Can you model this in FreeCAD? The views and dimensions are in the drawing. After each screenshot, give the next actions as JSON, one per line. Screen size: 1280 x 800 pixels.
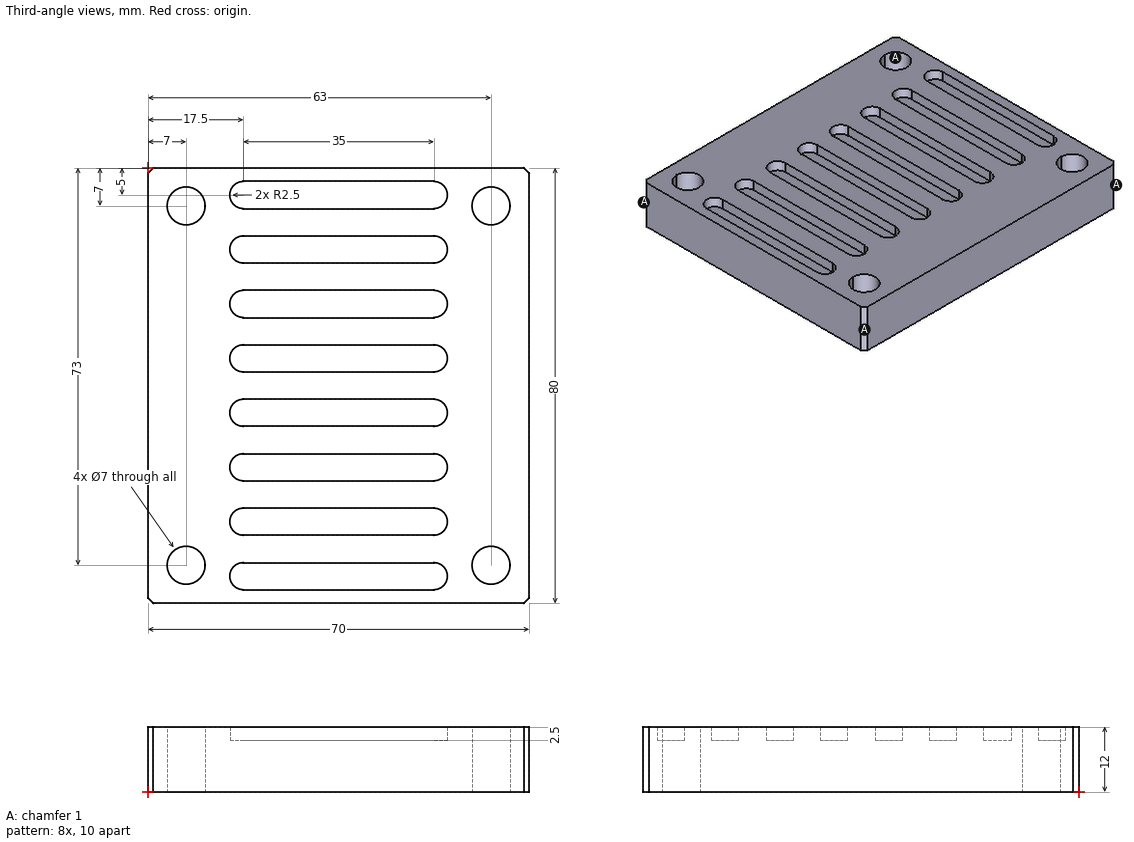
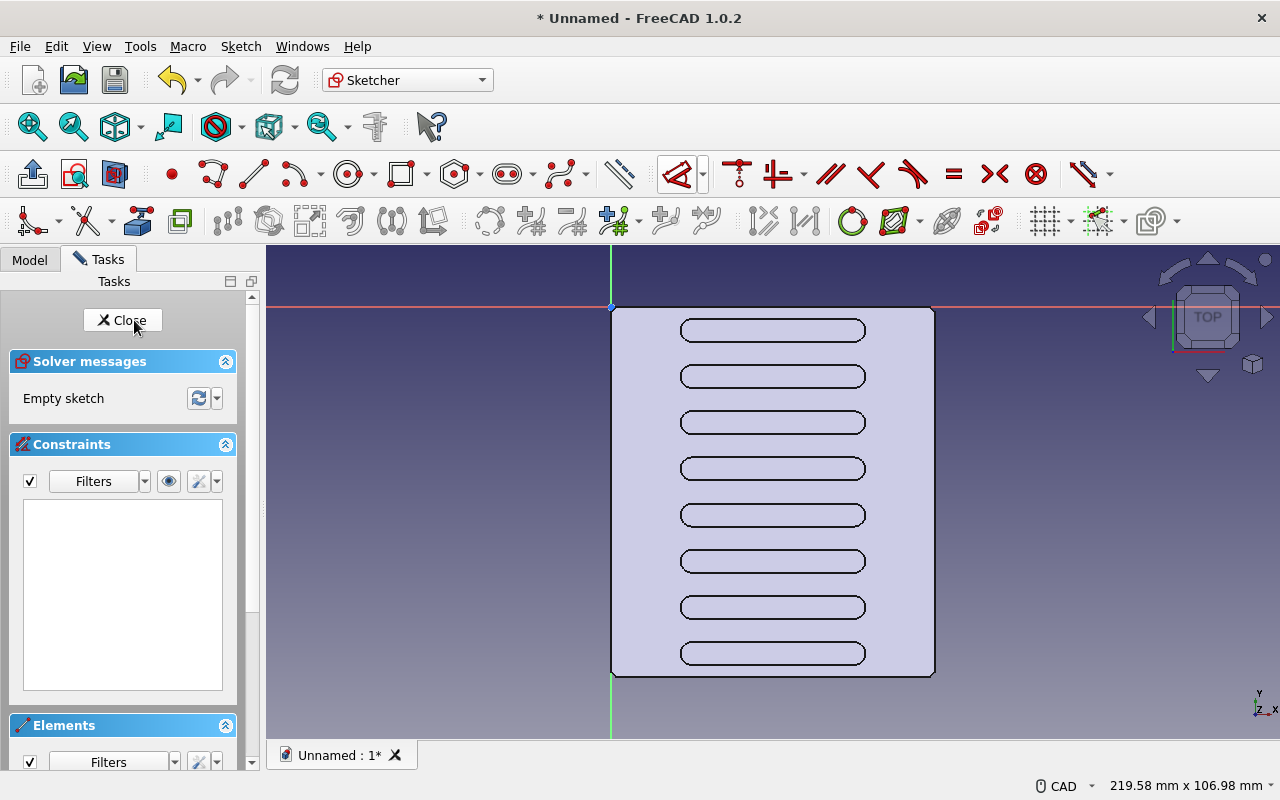
{"action": "key", "text": "q s"}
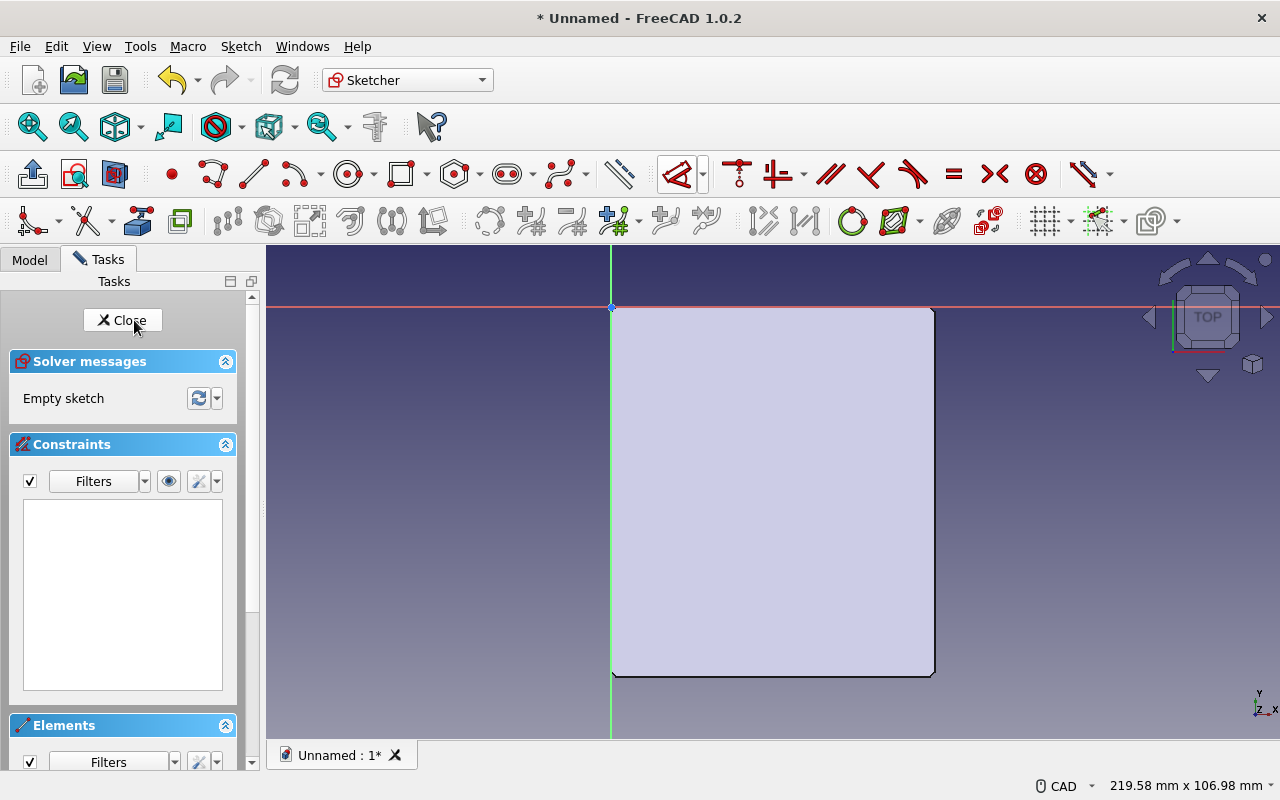
{"action": "left_click", "coordinate": [348, 174]}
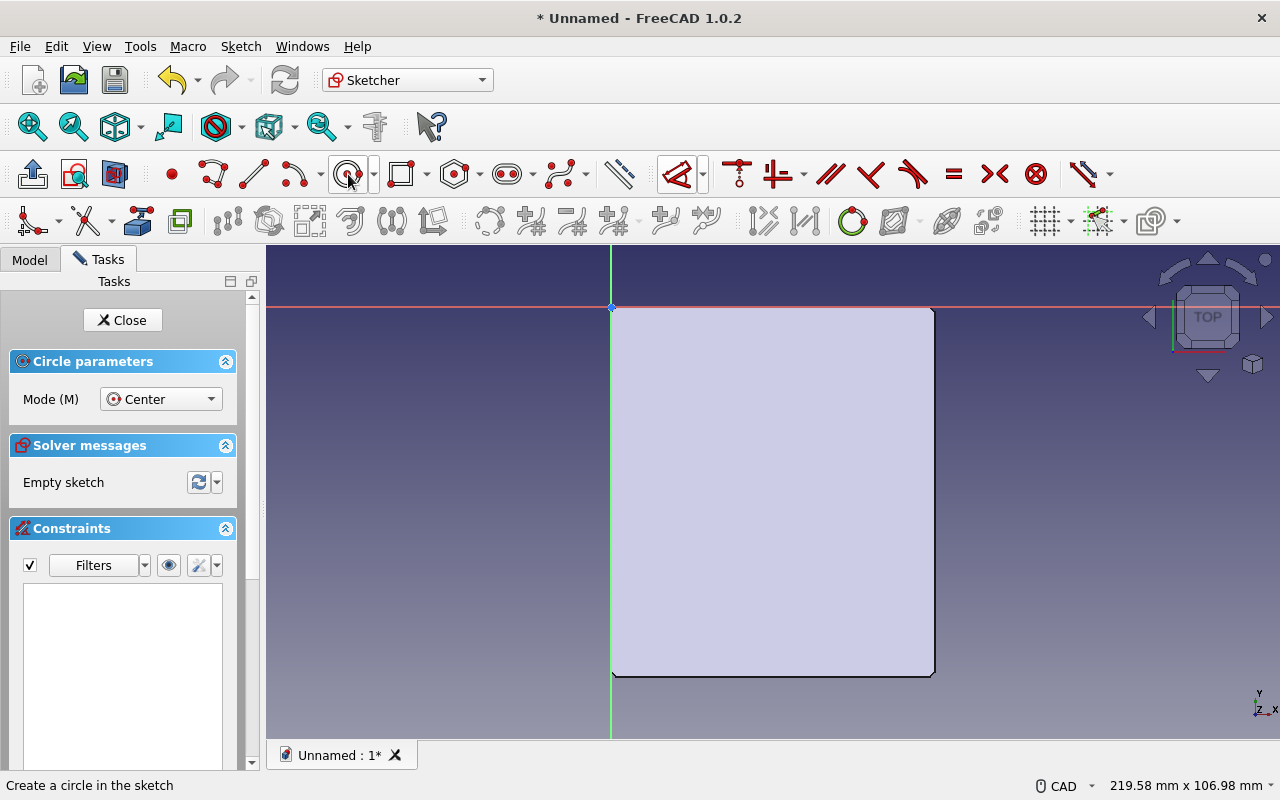
{"action": "scroll", "coordinate": [644, 644], "scroll_direction": "up", "scroll_amount": 2}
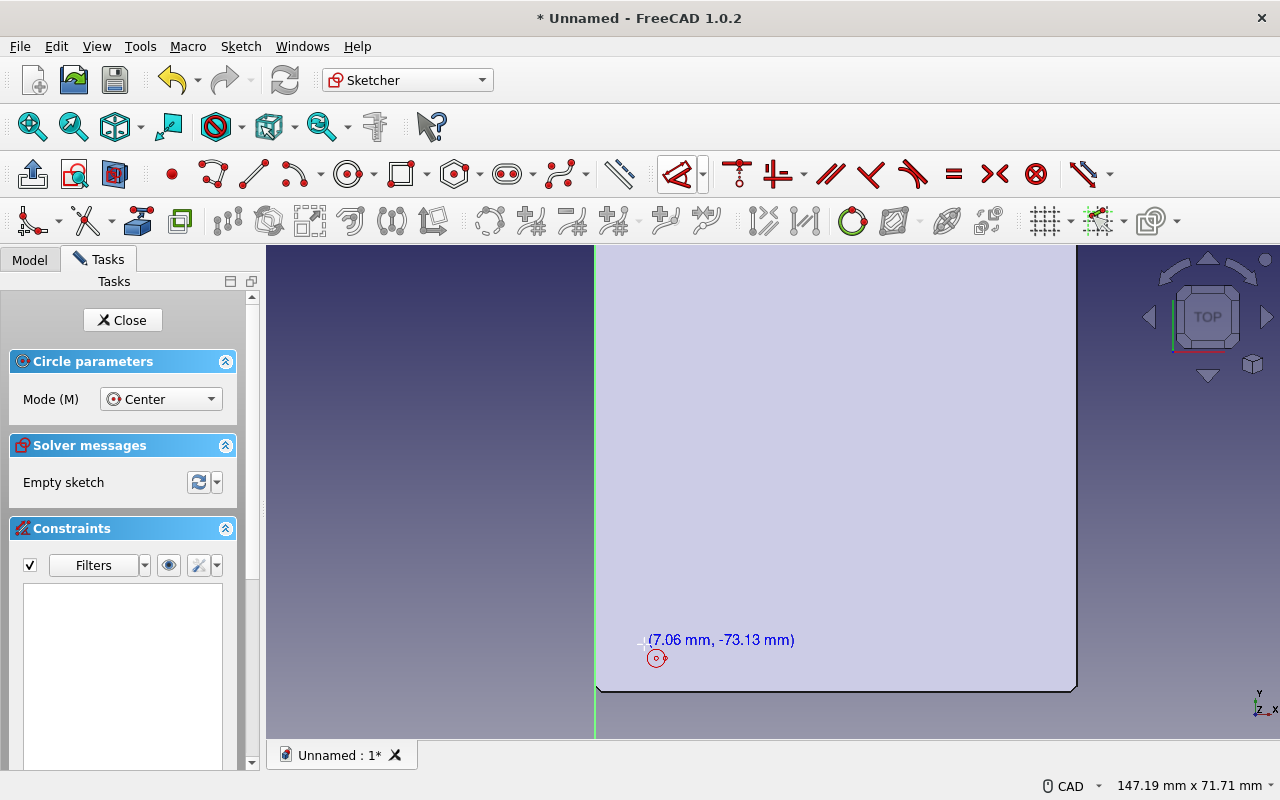
{"action": "left_click", "coordinate": [643, 644]}
{"action": "mouse_move", "coordinate": [660, 627]}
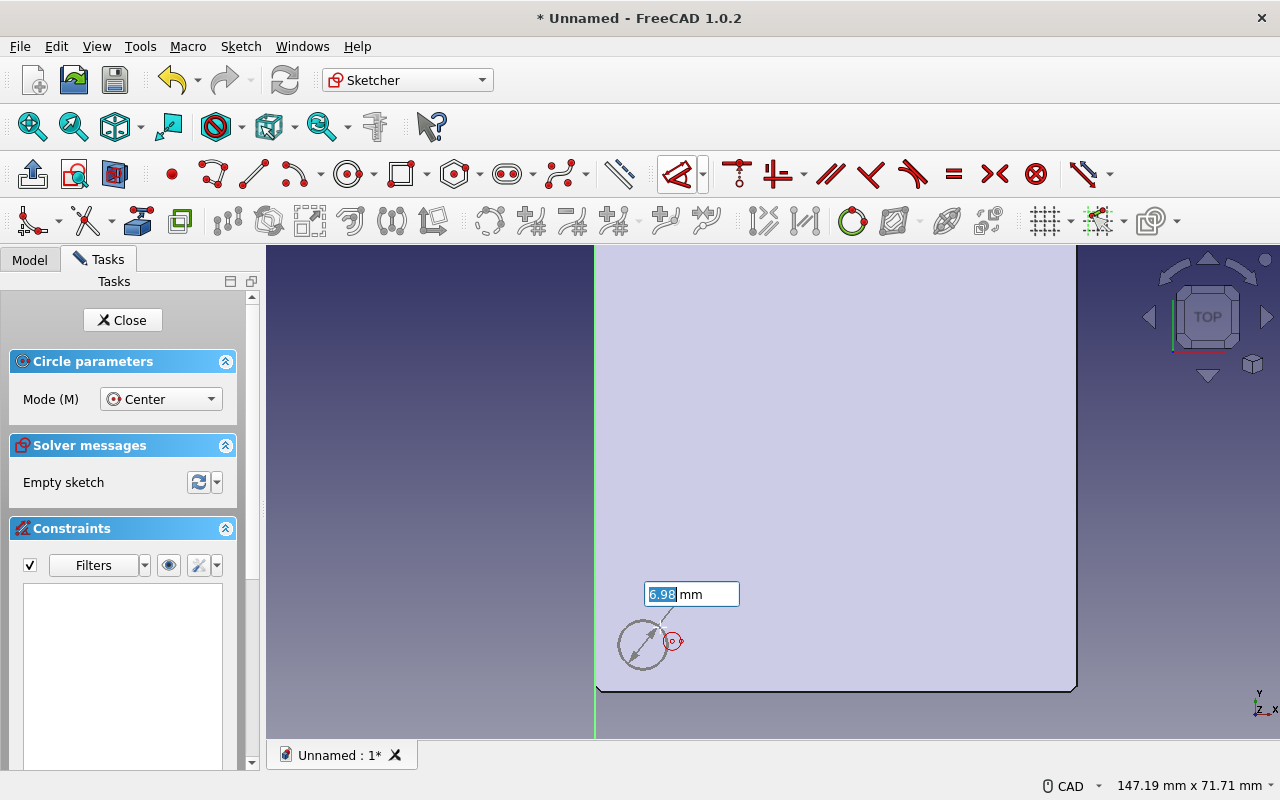
{"action": "type", "text": "7"}
{"action": "key", "text": "Return"}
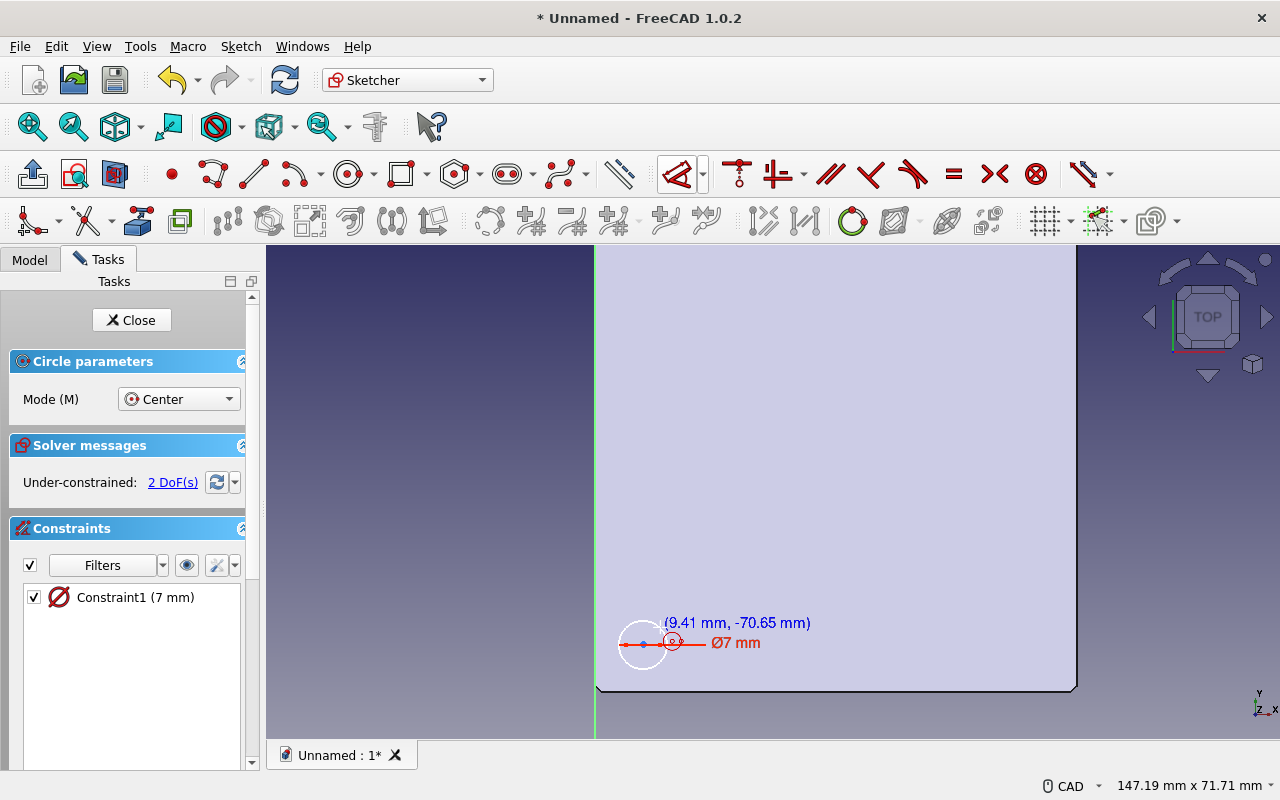
{"action": "scroll", "coordinate": [559, 598], "scroll_direction": "down", "scroll_amount": 3}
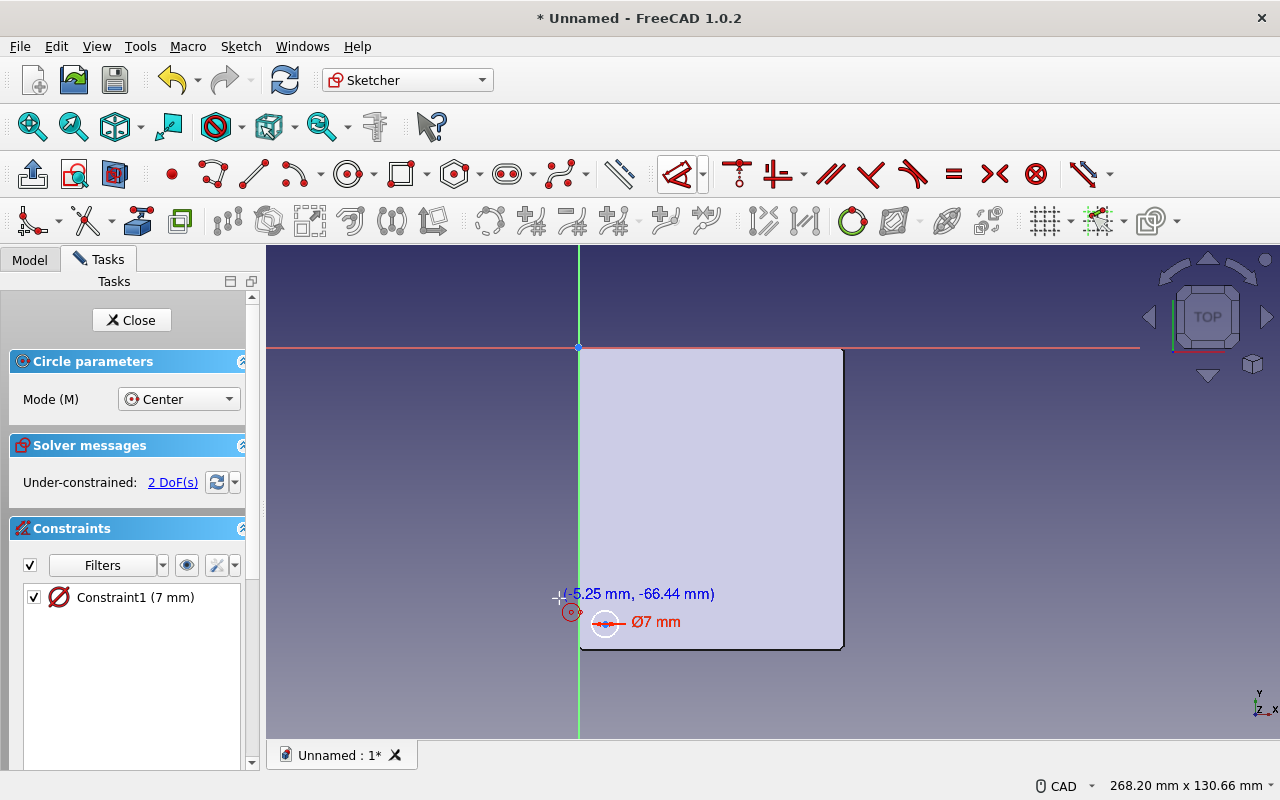
{"action": "scroll", "coordinate": [605, 374], "scroll_direction": "up", "scroll_amount": 3}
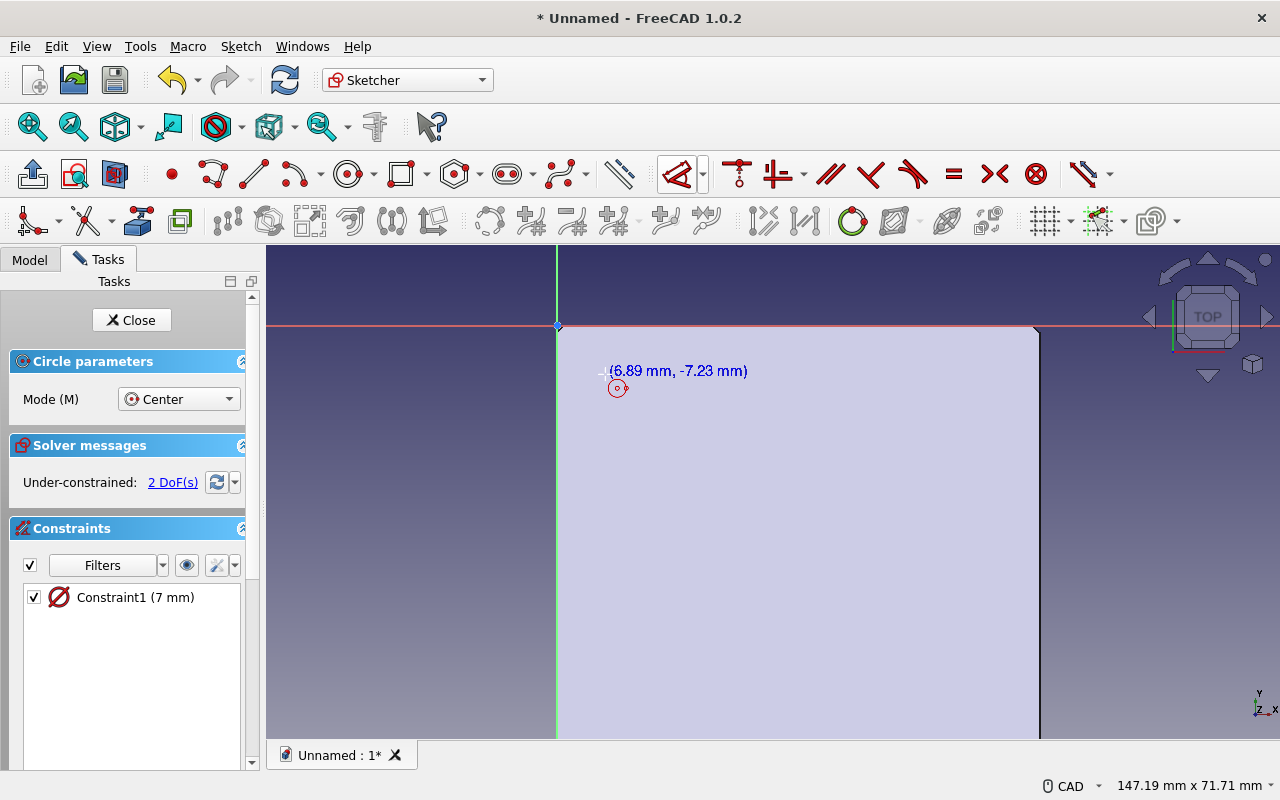
{"action": "left_click", "coordinate": [606, 374]}
{"action": "mouse_move", "coordinate": [623, 357]}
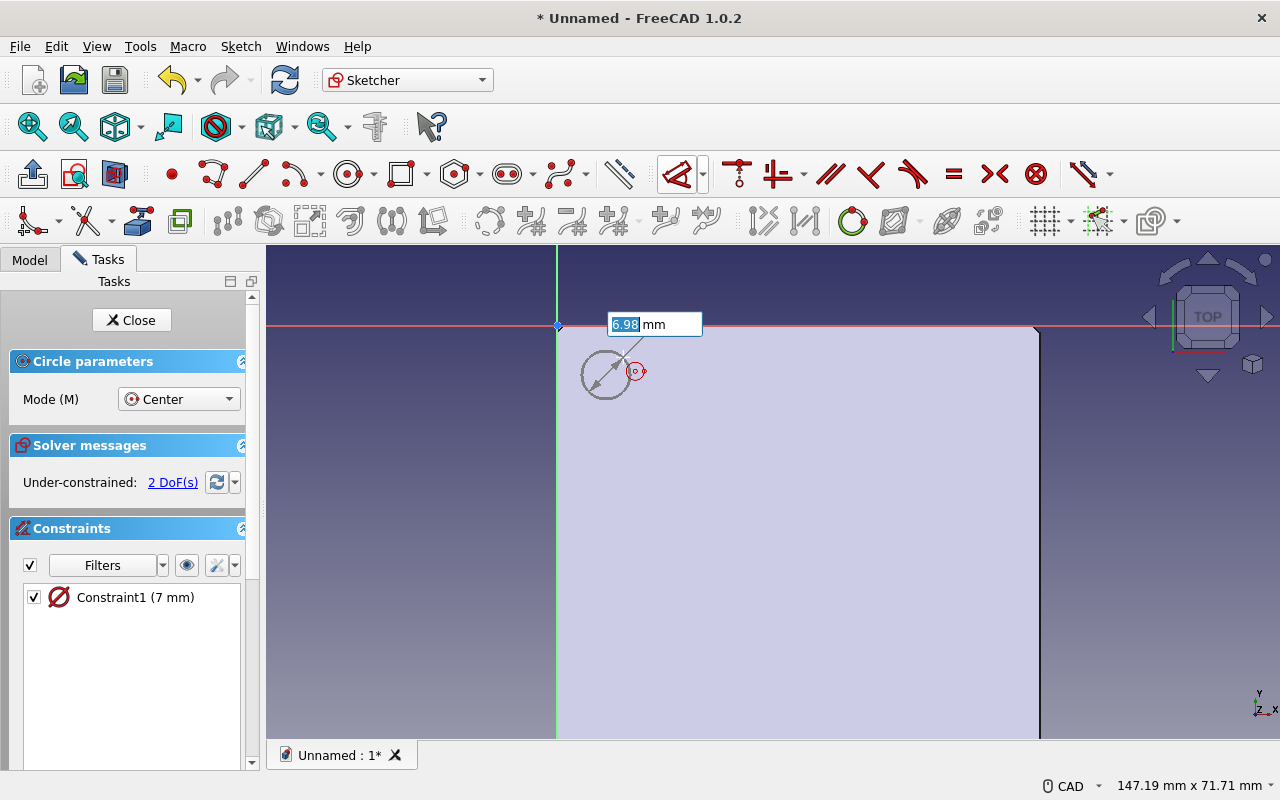
{"action": "type", "text": "7"}
{"action": "key", "text": "Return"}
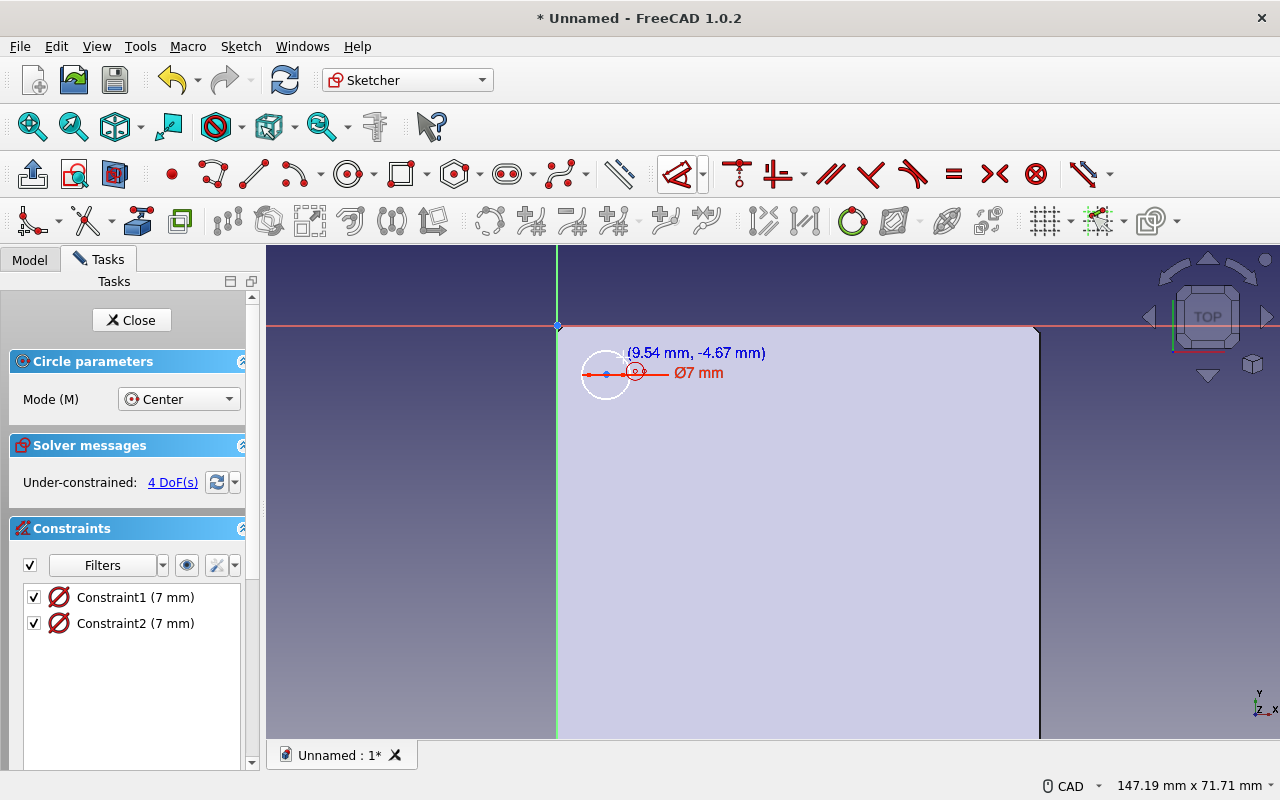
{"action": "scroll", "coordinate": [605, 374], "scroll_direction": "down", "scroll_amount": 3}